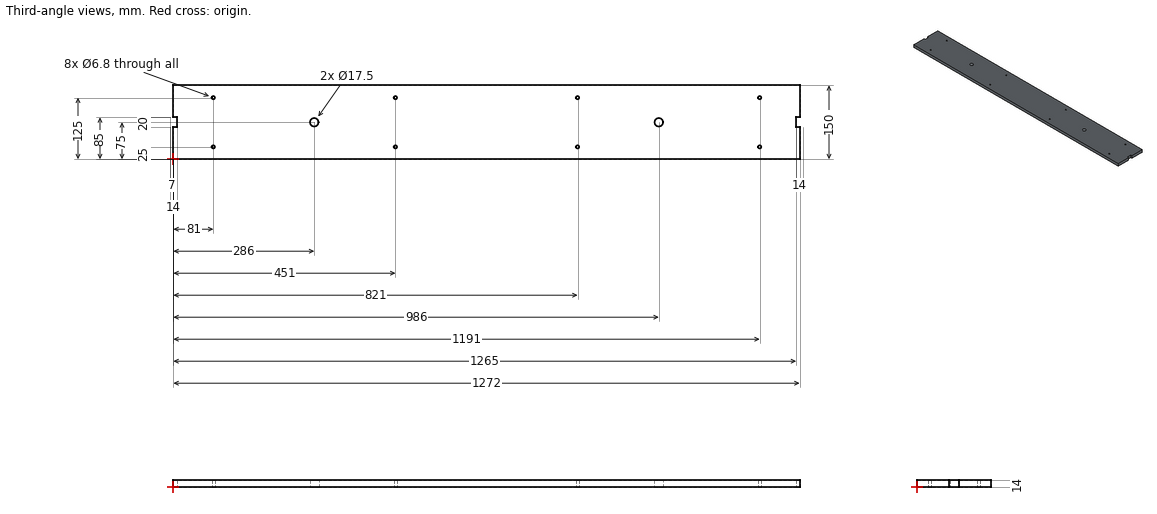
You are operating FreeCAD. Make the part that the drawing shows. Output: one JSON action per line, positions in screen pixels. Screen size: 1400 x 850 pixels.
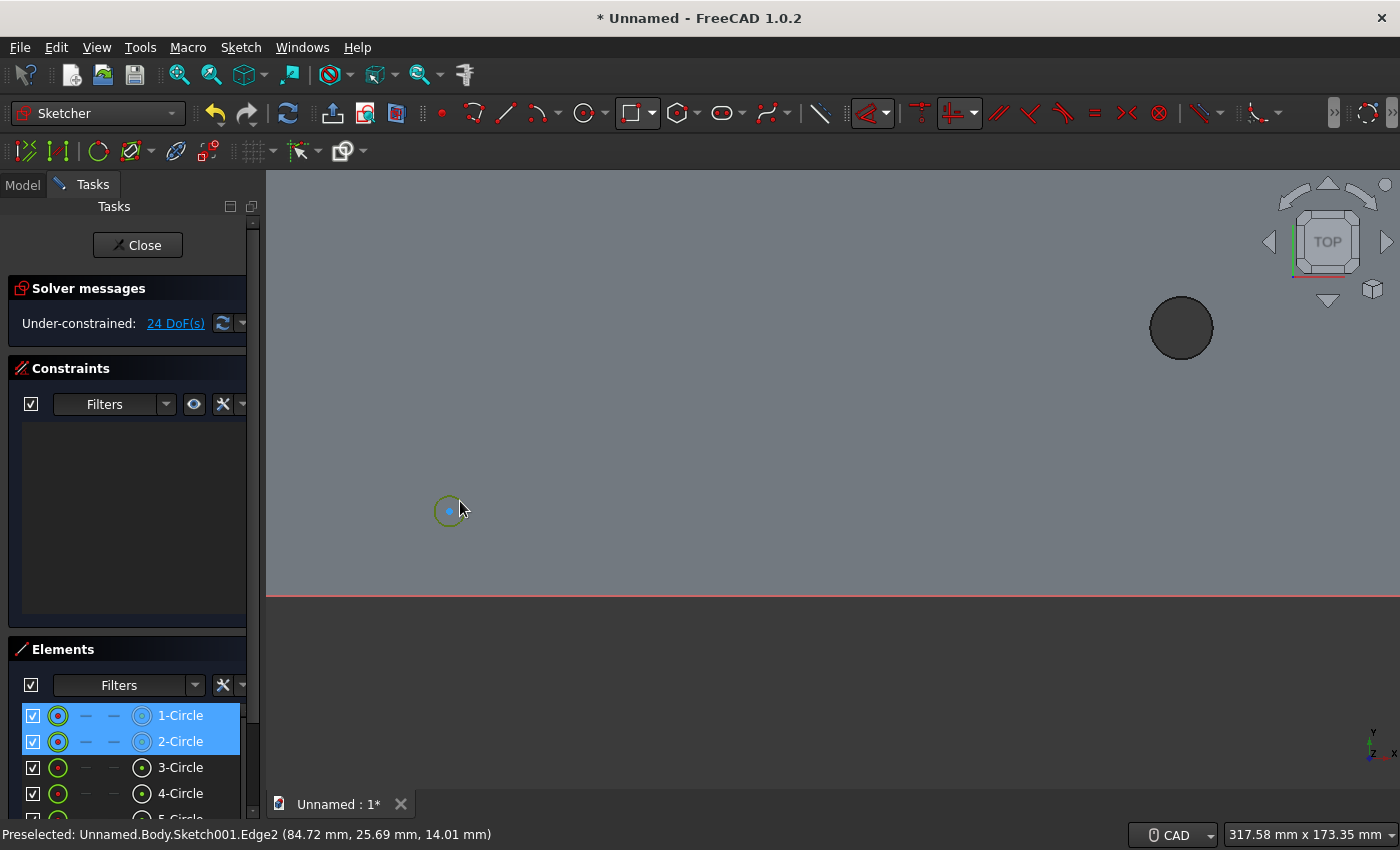
{"action": "scroll", "coordinate": [462, 502], "scroll_direction": "down", "scroll_amount": 9}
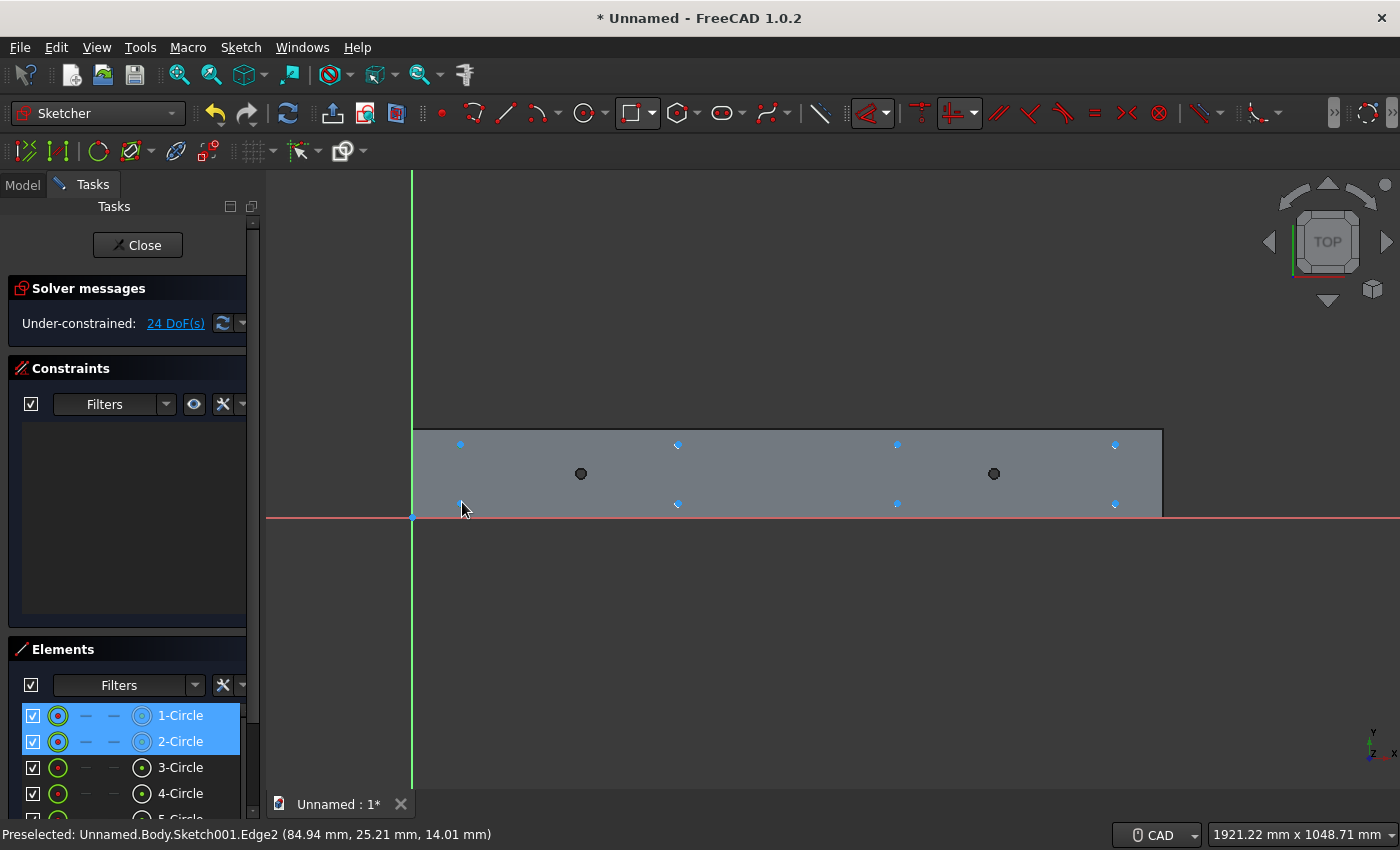
{"action": "scroll", "coordinate": [680, 443], "scroll_direction": "up", "scroll_amount": 8}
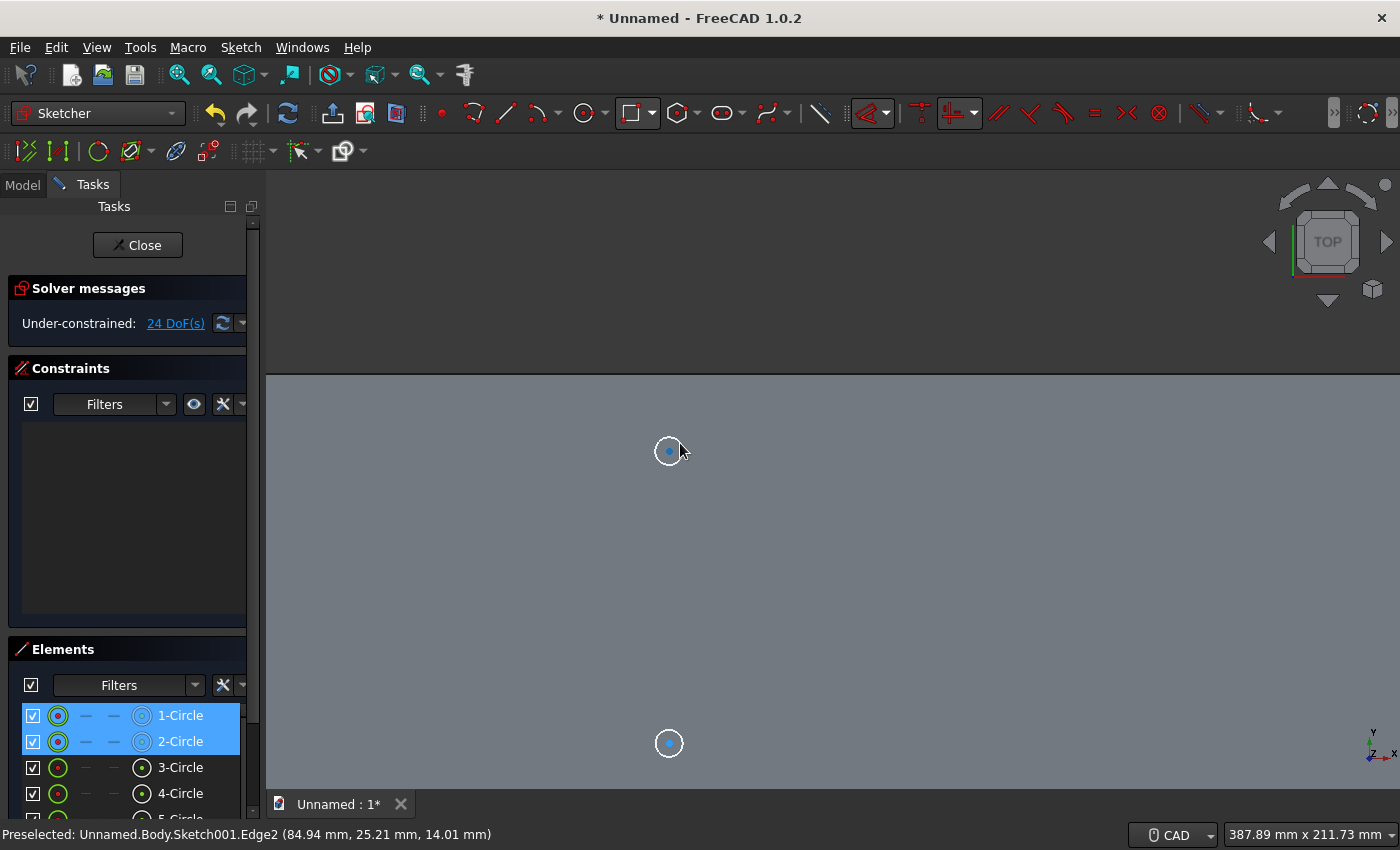
{"action": "left_click", "coordinate": [679, 441]}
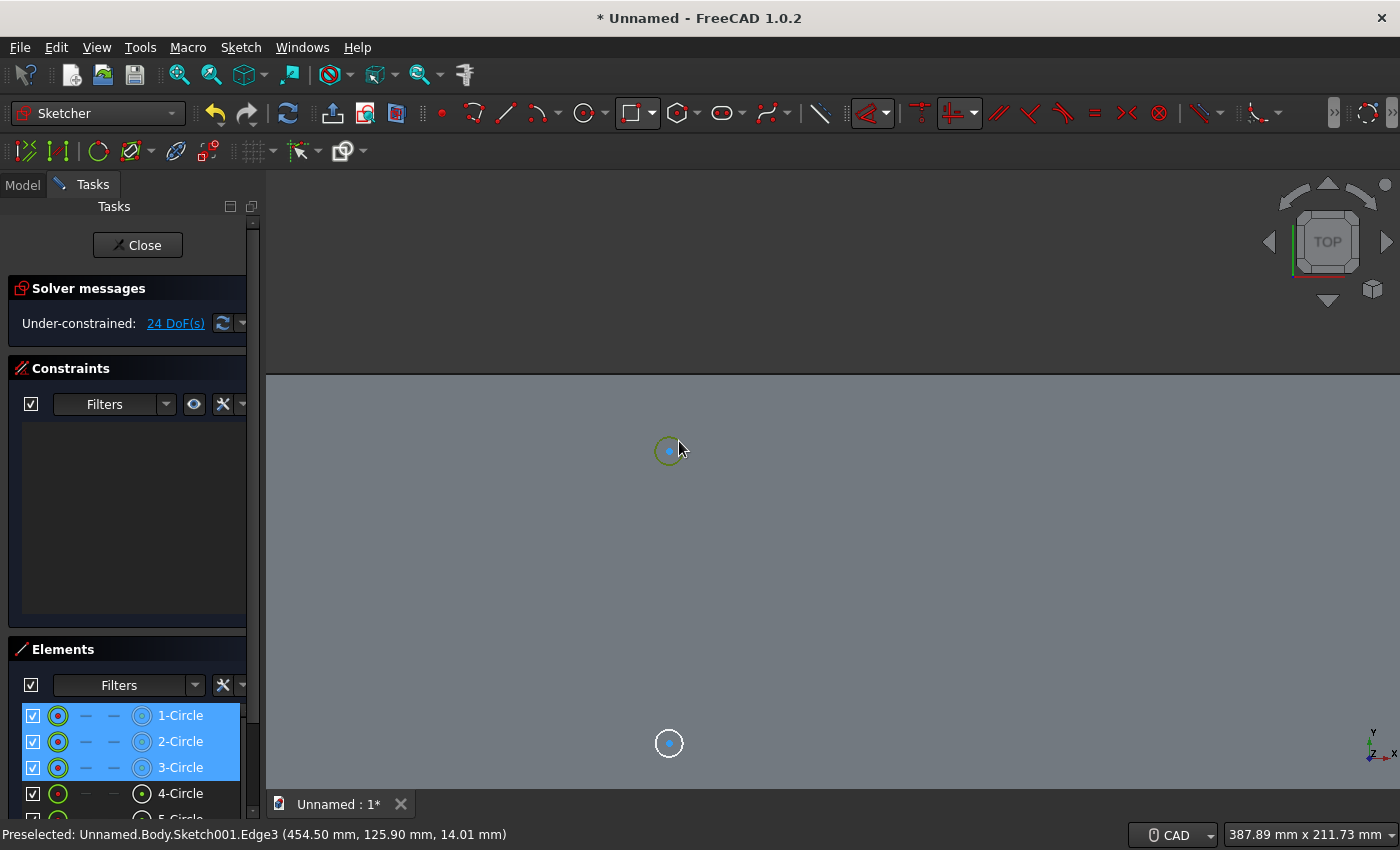
{"action": "left_click", "coordinate": [679, 734]}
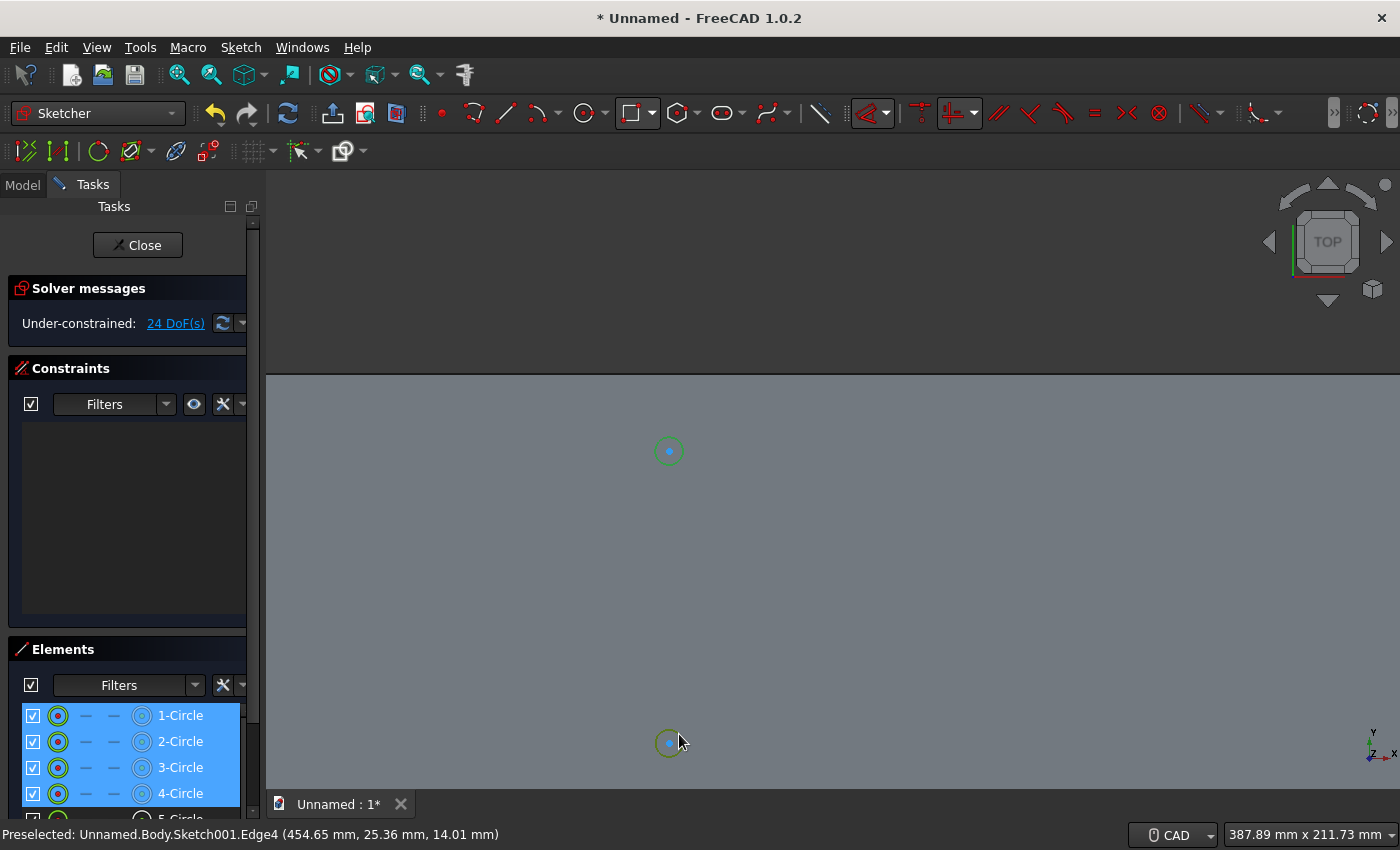
{"action": "scroll", "coordinate": [680, 443], "scroll_direction": "down", "scroll_amount": 8}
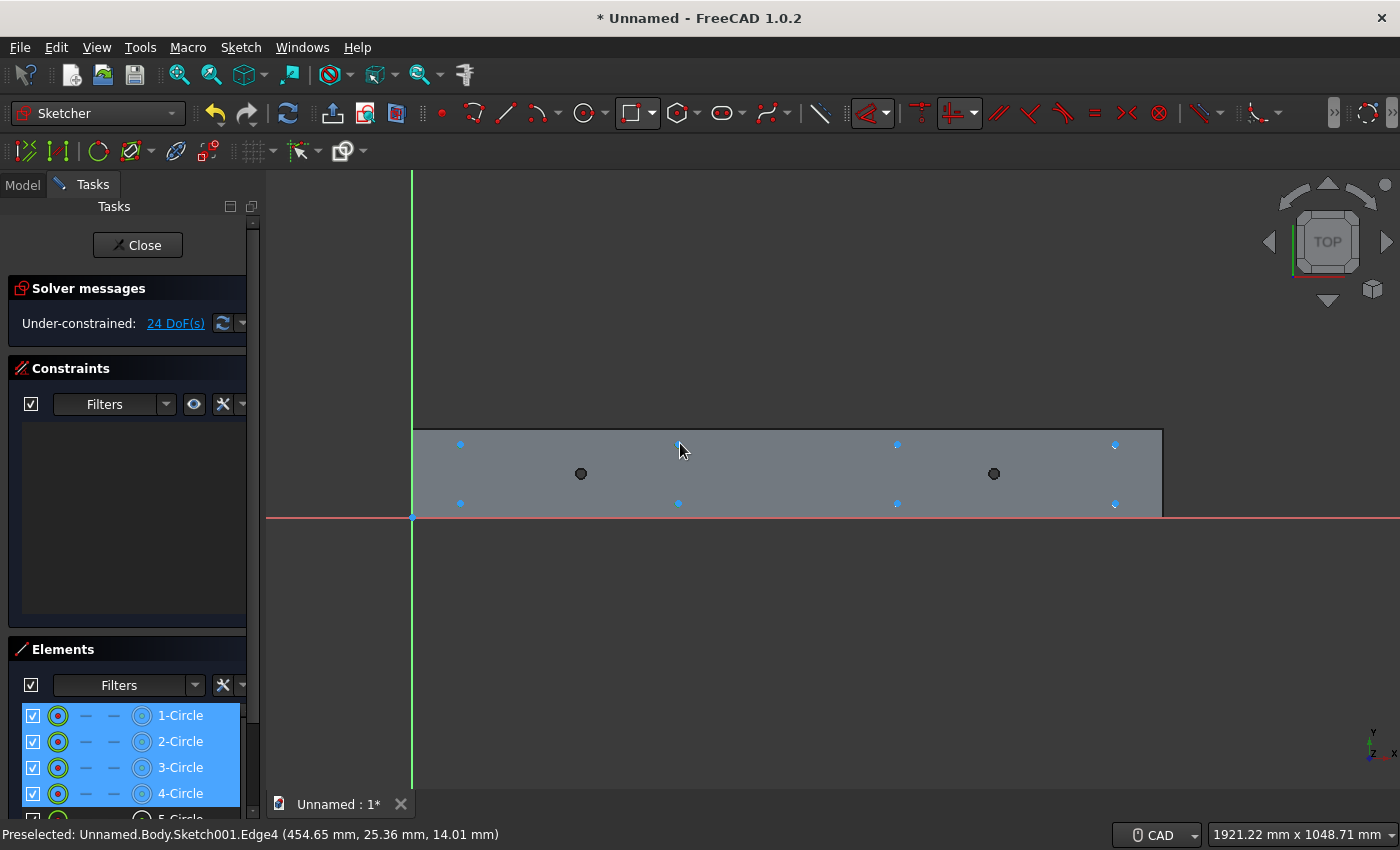
{"action": "scroll", "coordinate": [899, 443], "scroll_direction": "up", "scroll_amount": 9}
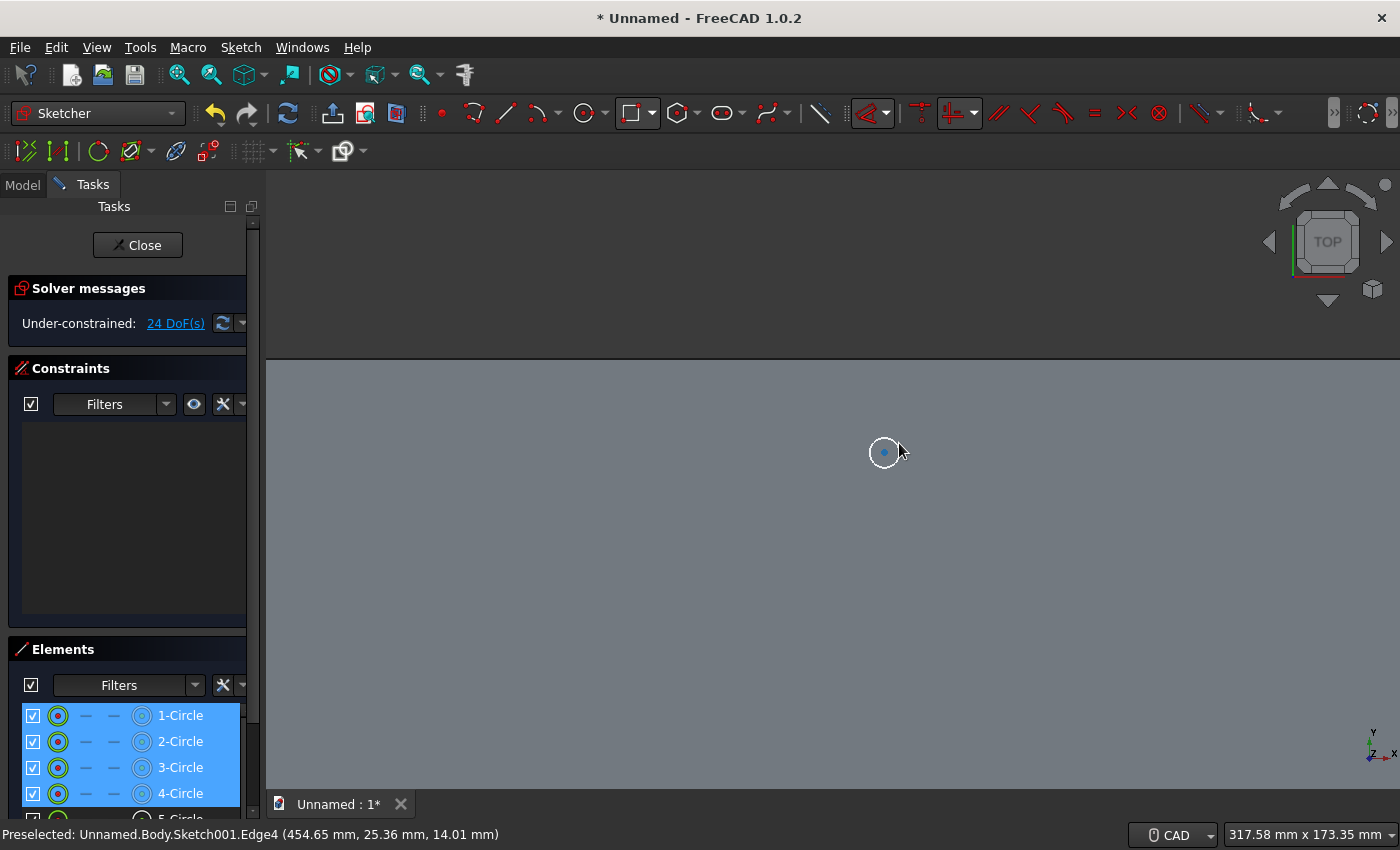
{"action": "left_click", "coordinate": [895, 442]}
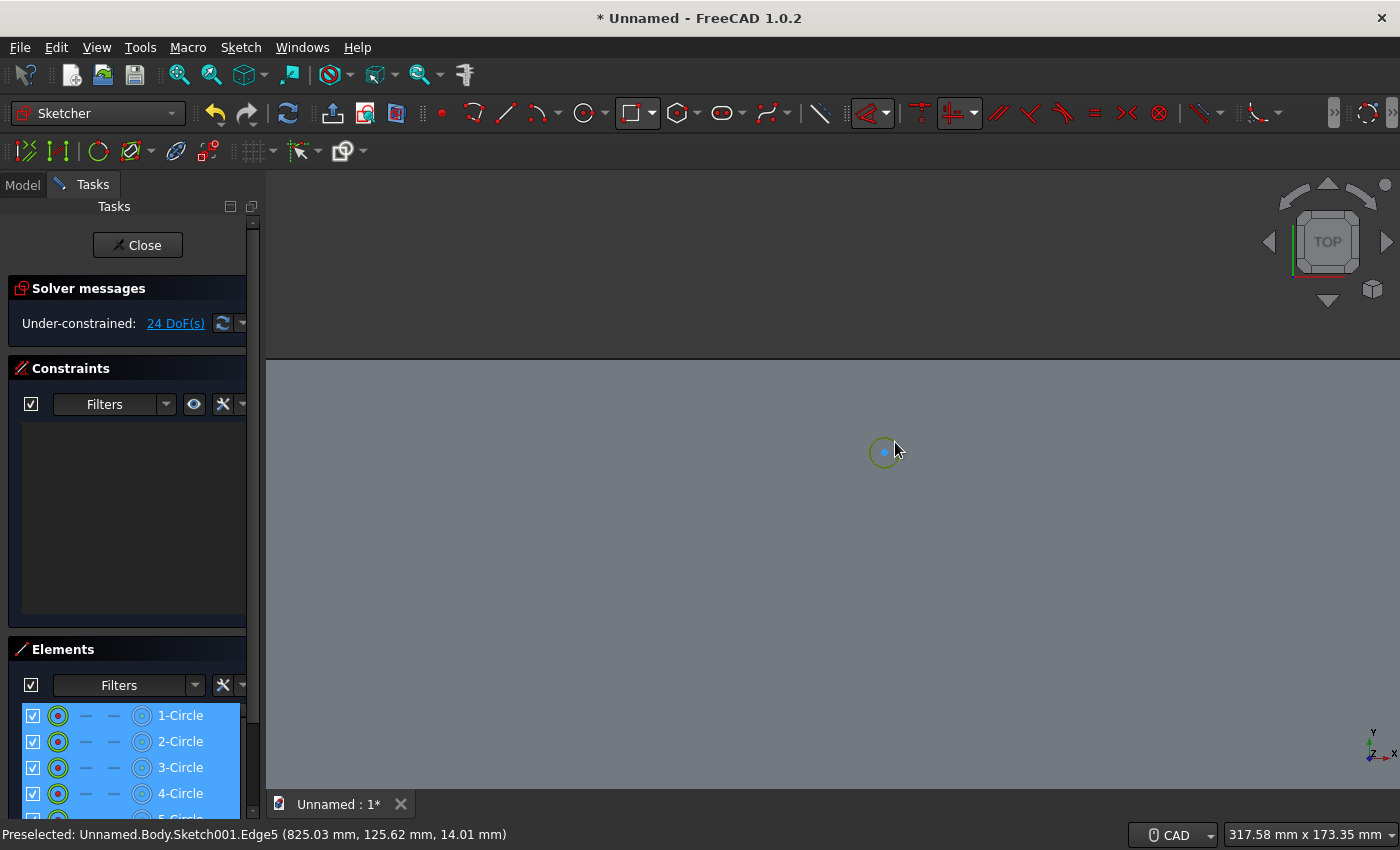
{"action": "scroll", "coordinate": [899, 443], "scroll_direction": "down", "scroll_amount": 9}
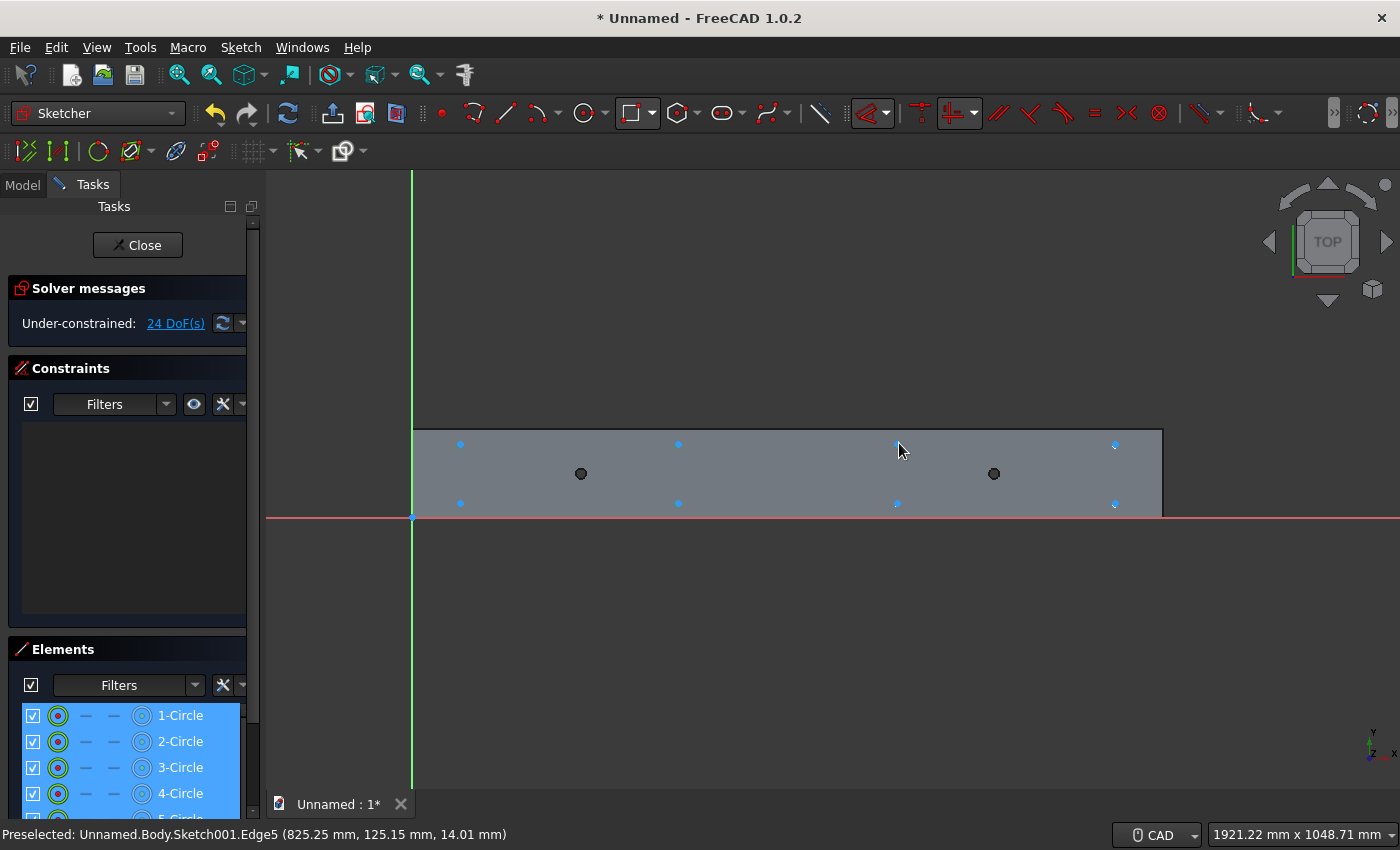
{"action": "scroll", "coordinate": [899, 502], "scroll_direction": "up", "scroll_amount": 9}